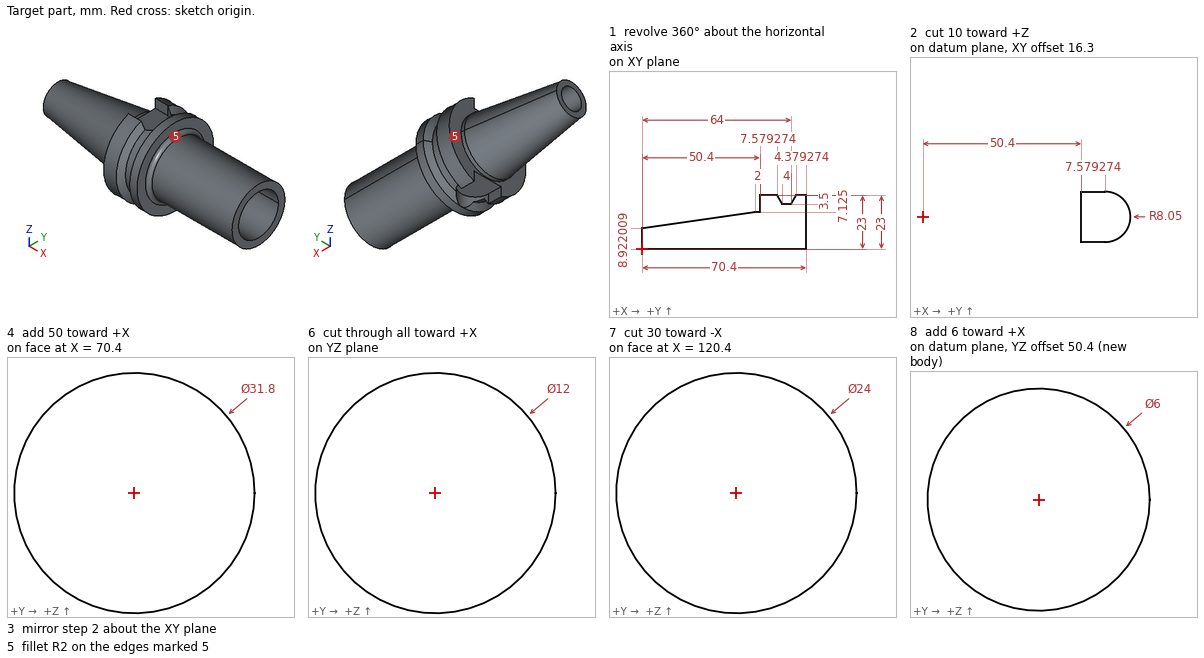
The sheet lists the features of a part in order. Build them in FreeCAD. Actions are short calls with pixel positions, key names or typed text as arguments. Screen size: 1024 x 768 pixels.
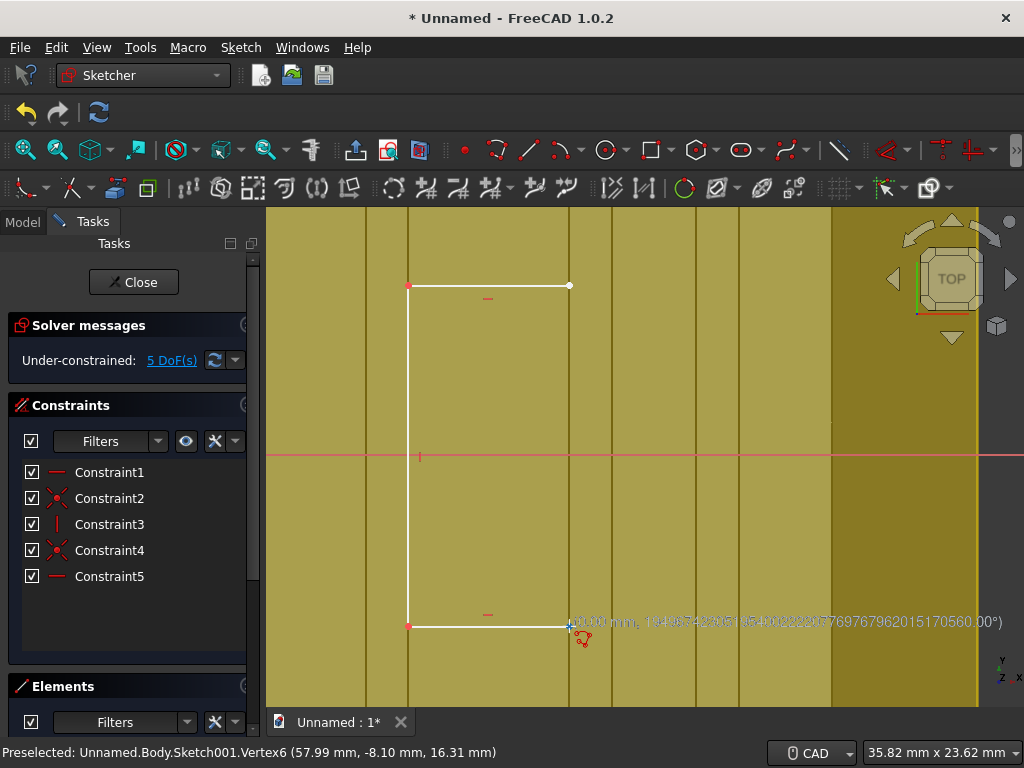
click(584, 150)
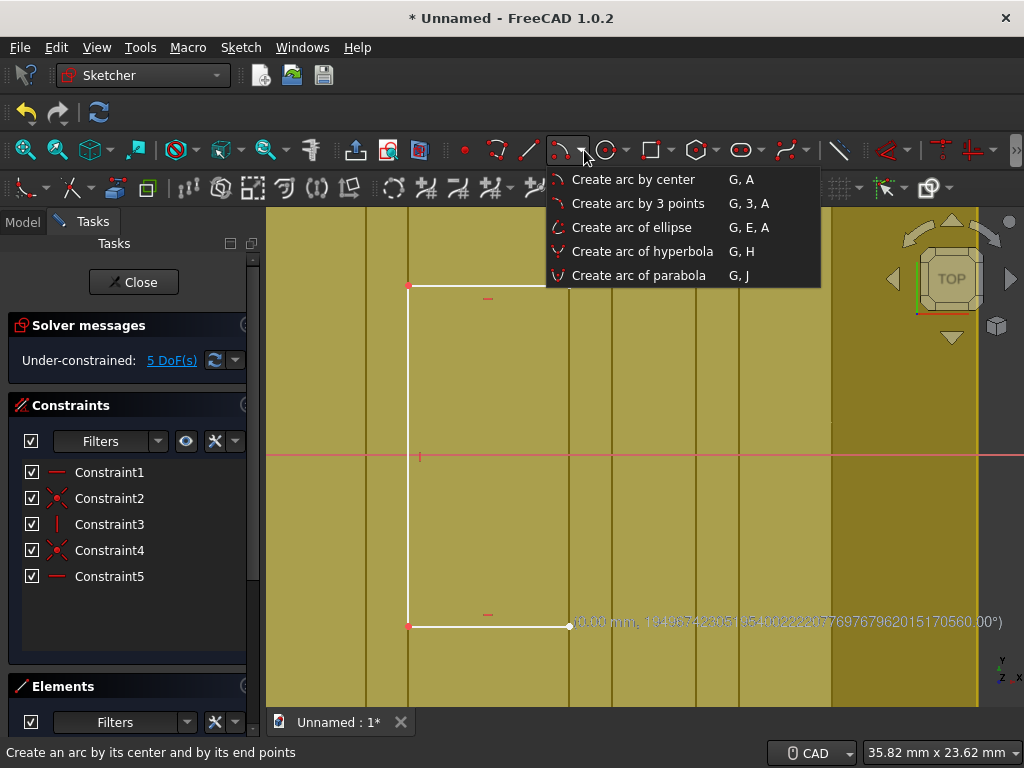
click(684, 203)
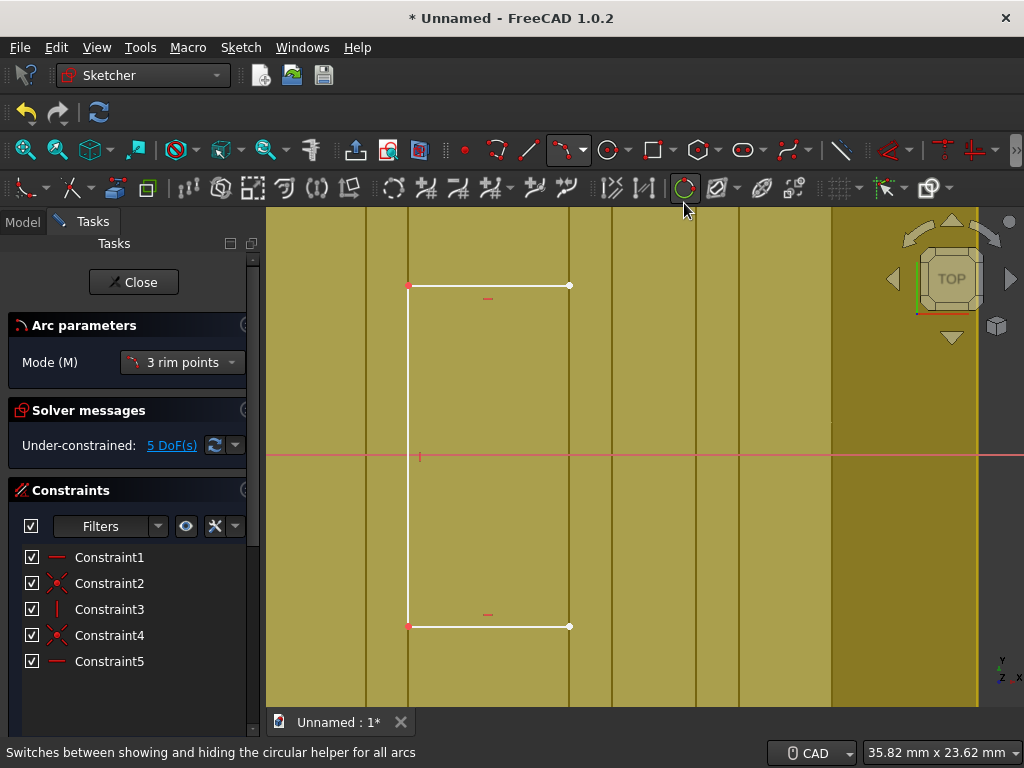
click(569, 627)
click(569, 286)
click(731, 508)
key(Escape)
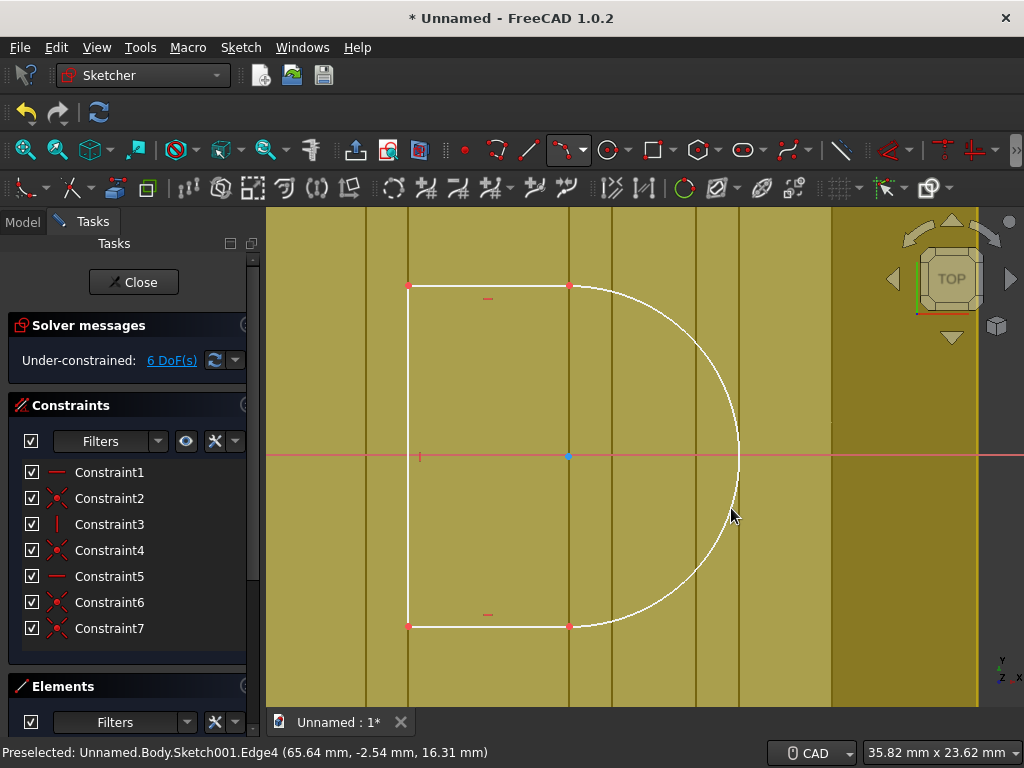
click(521, 286)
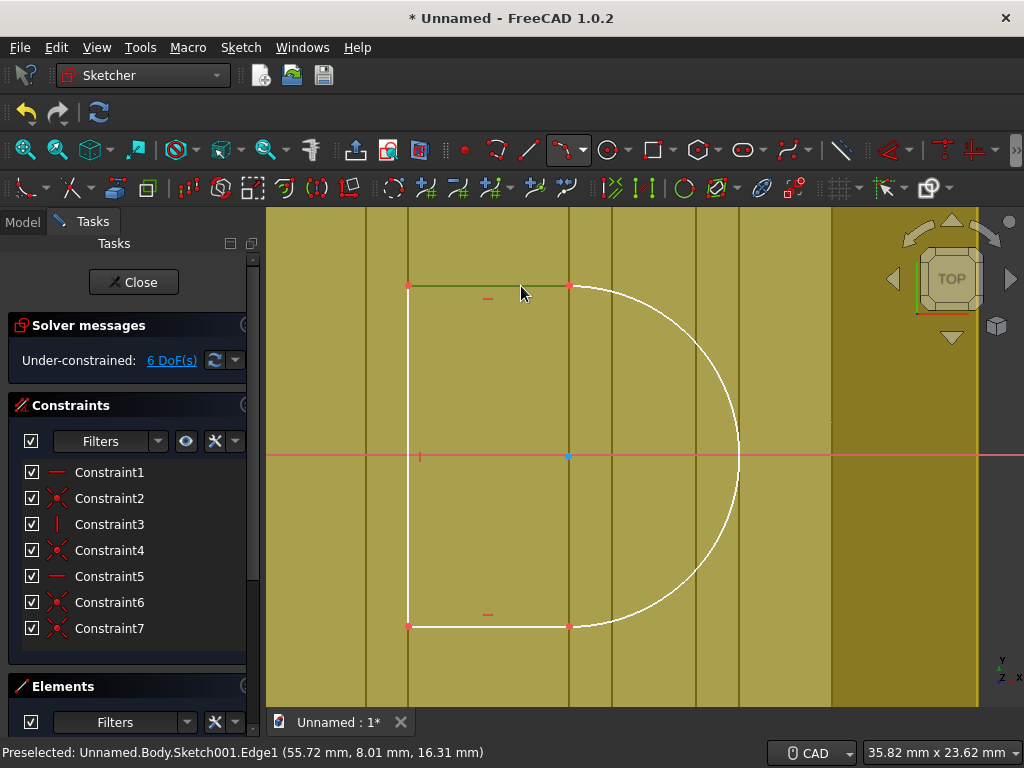
click(707, 557)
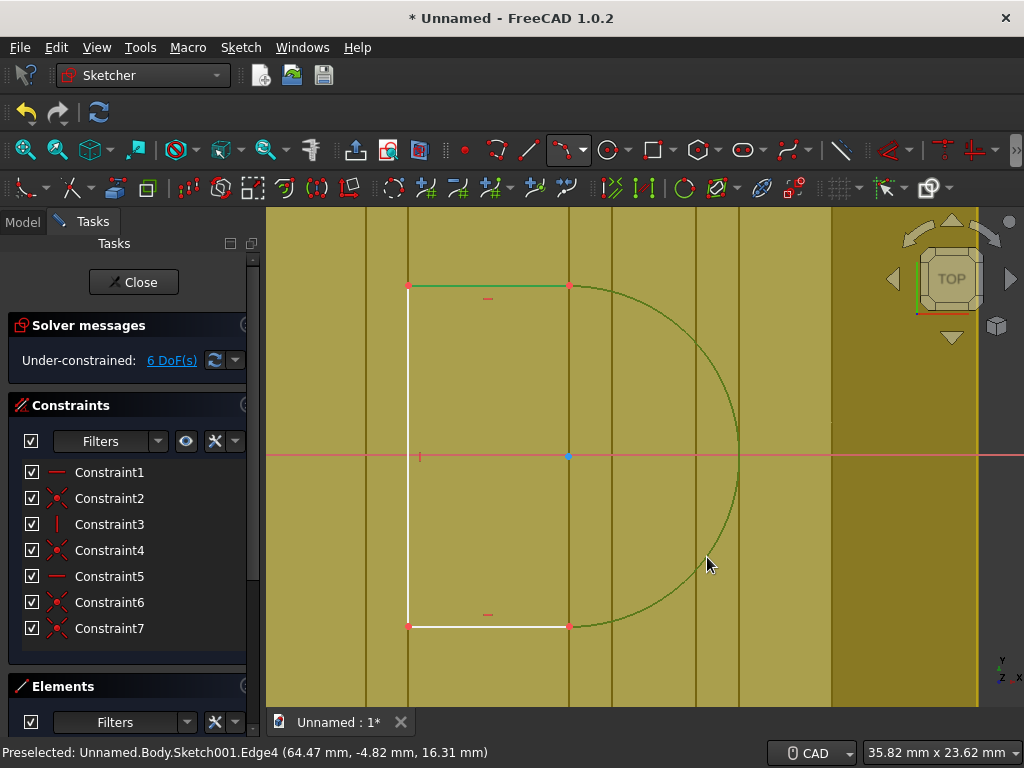
key(t)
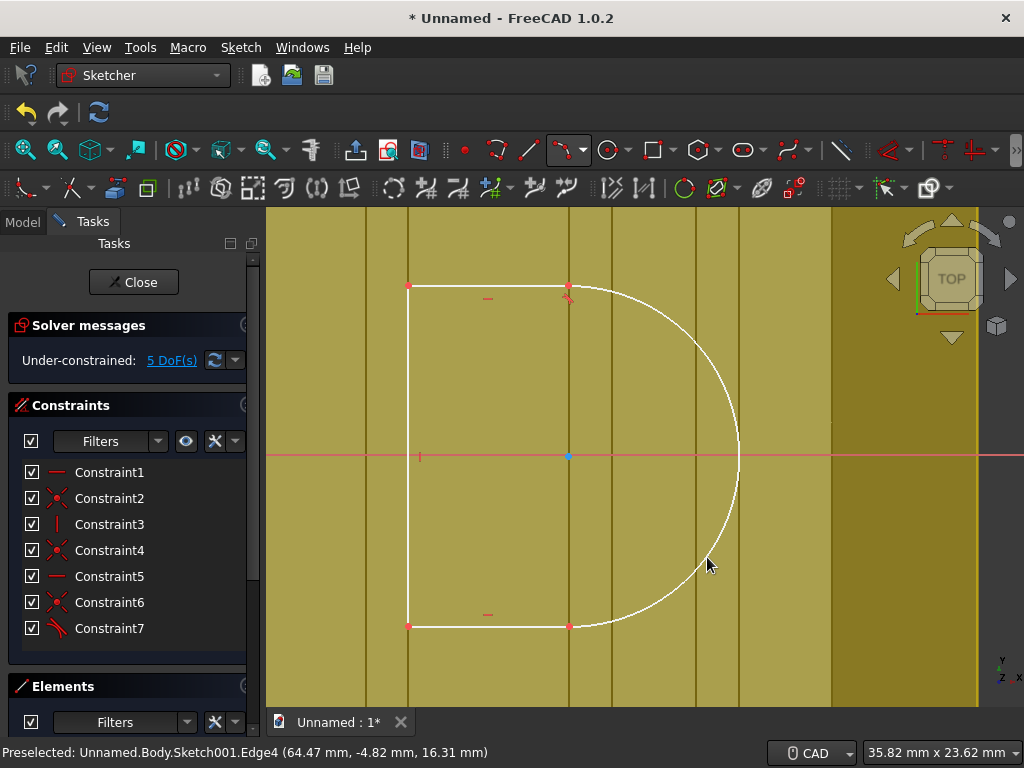
click(456, 627)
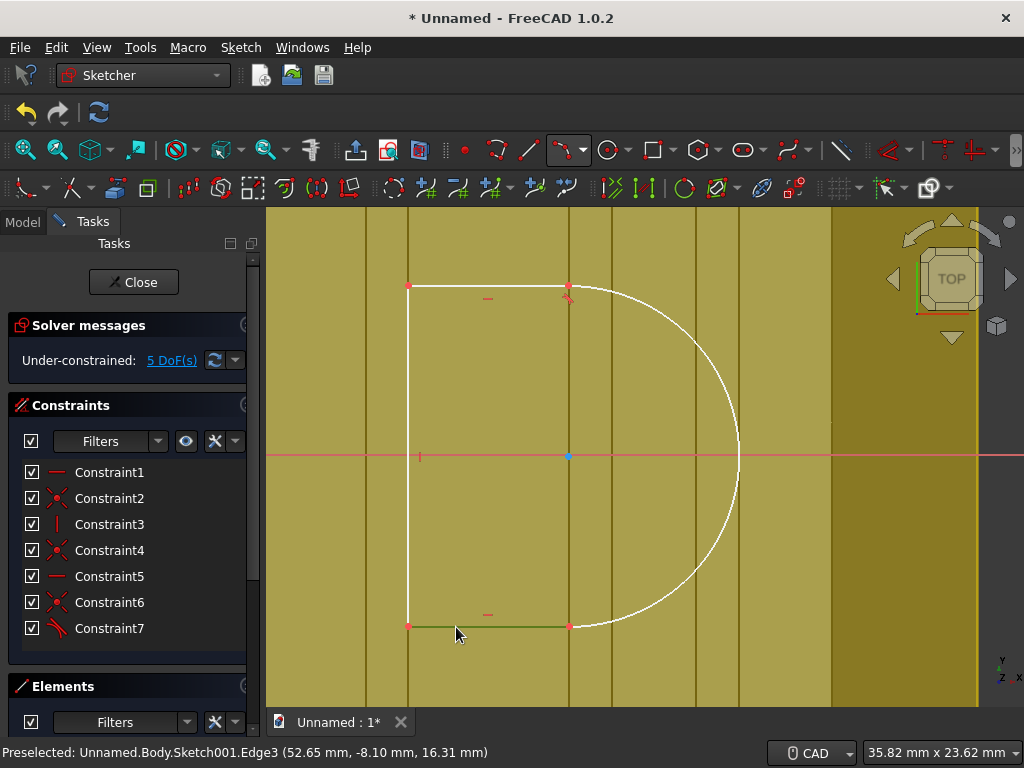
click(707, 557)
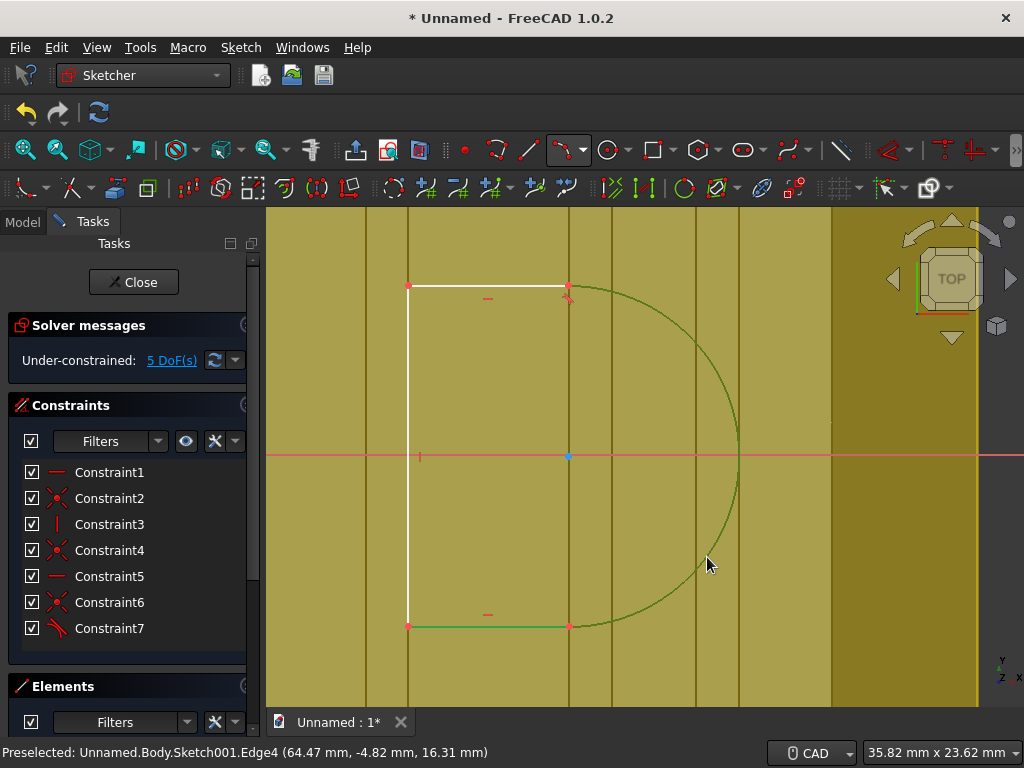
key(t)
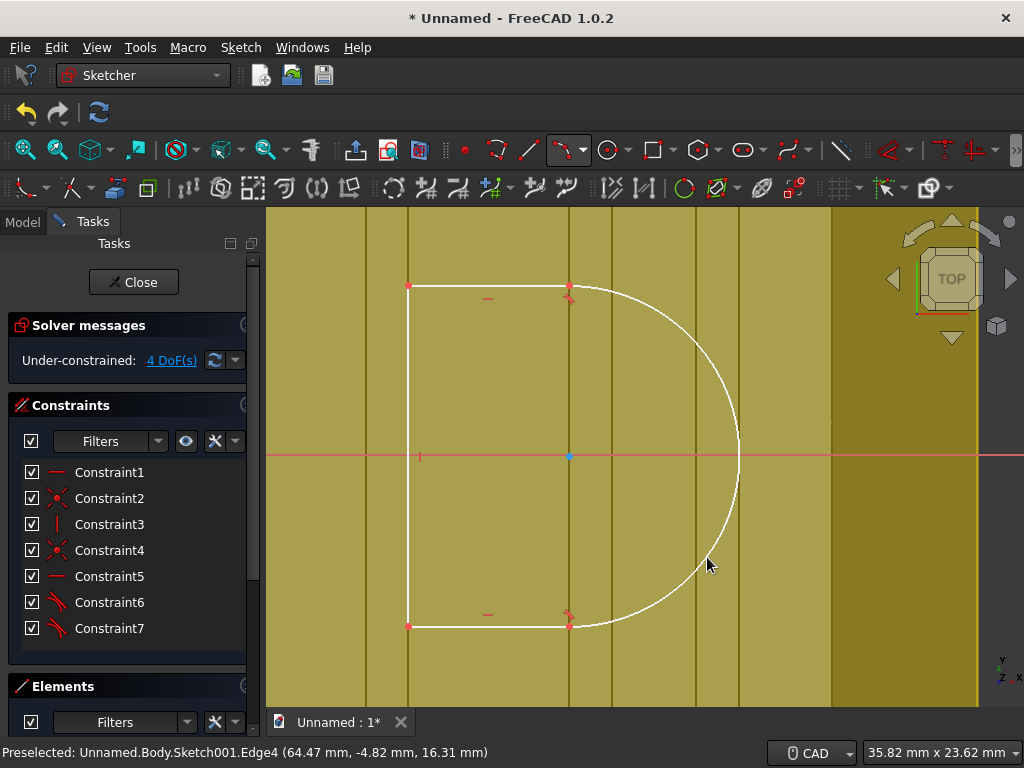
click(569, 457)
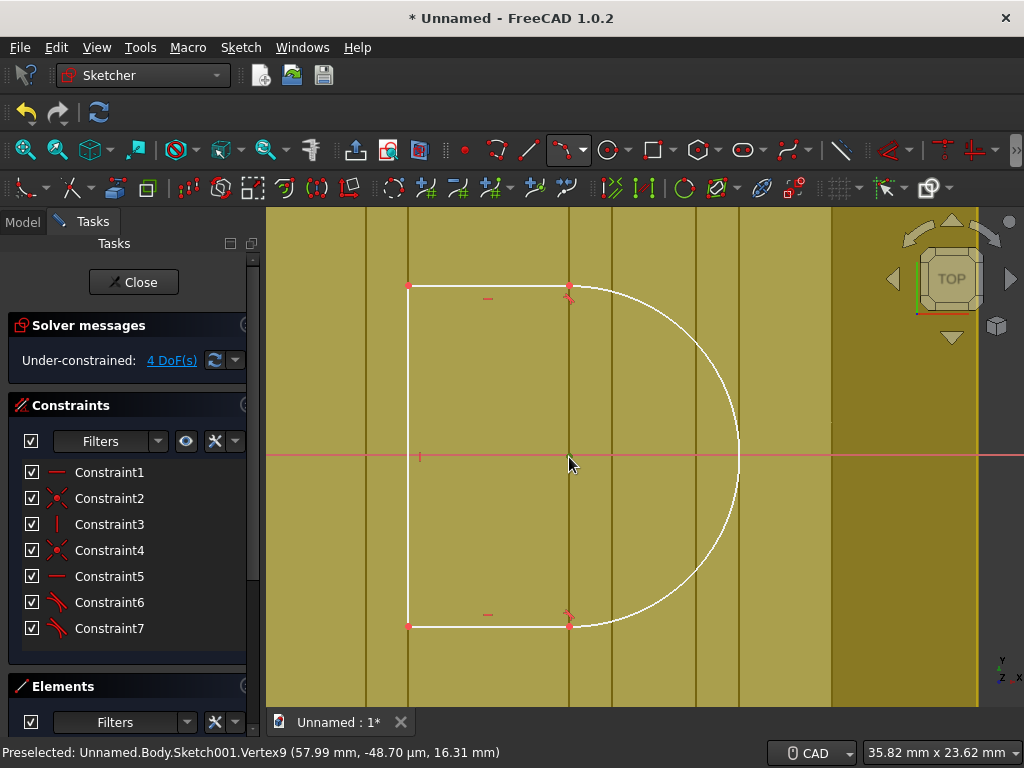
click(334, 455)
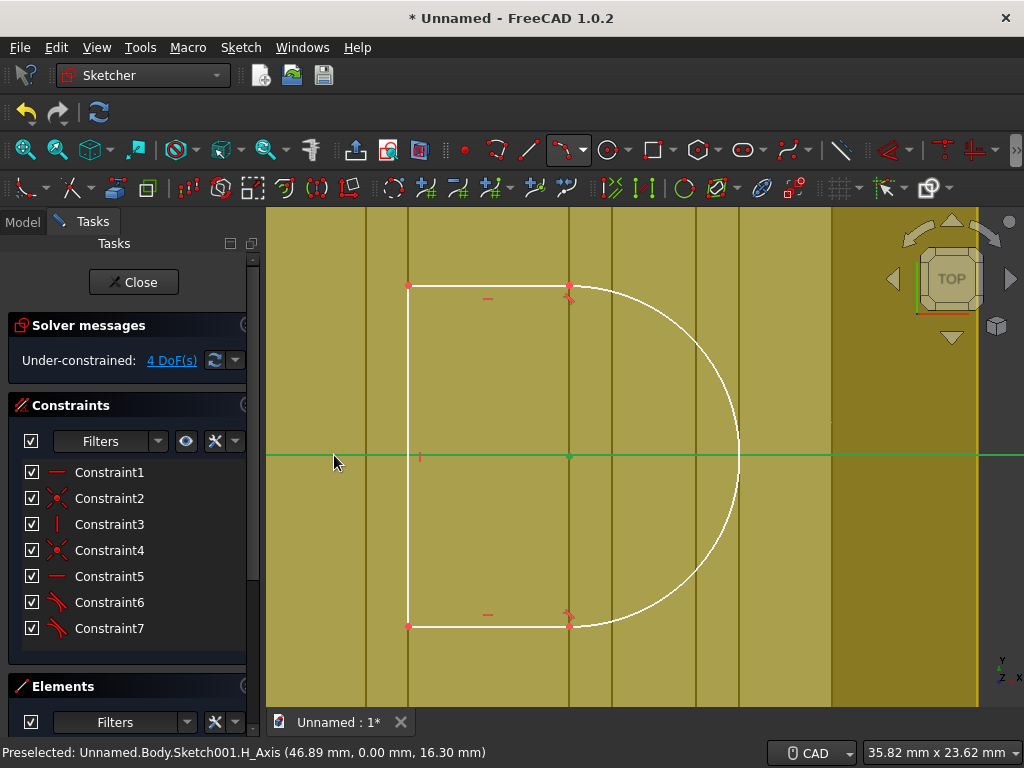
click(944, 150)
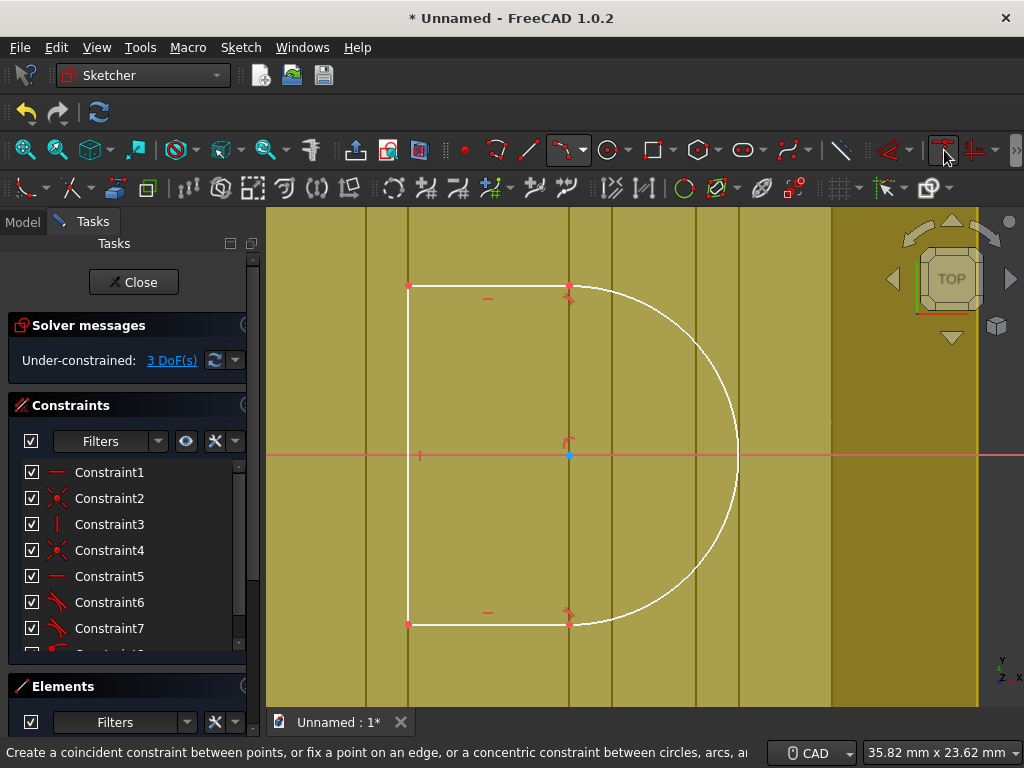
key(d)